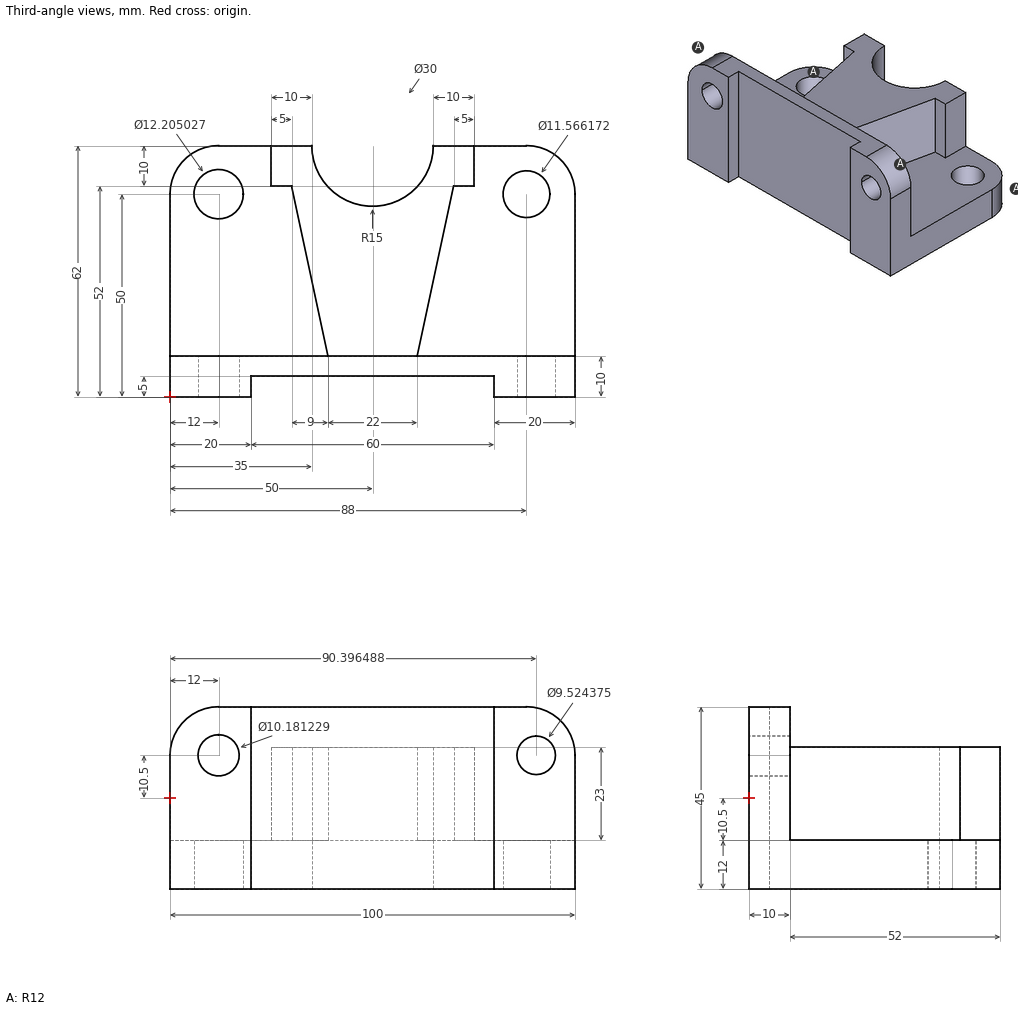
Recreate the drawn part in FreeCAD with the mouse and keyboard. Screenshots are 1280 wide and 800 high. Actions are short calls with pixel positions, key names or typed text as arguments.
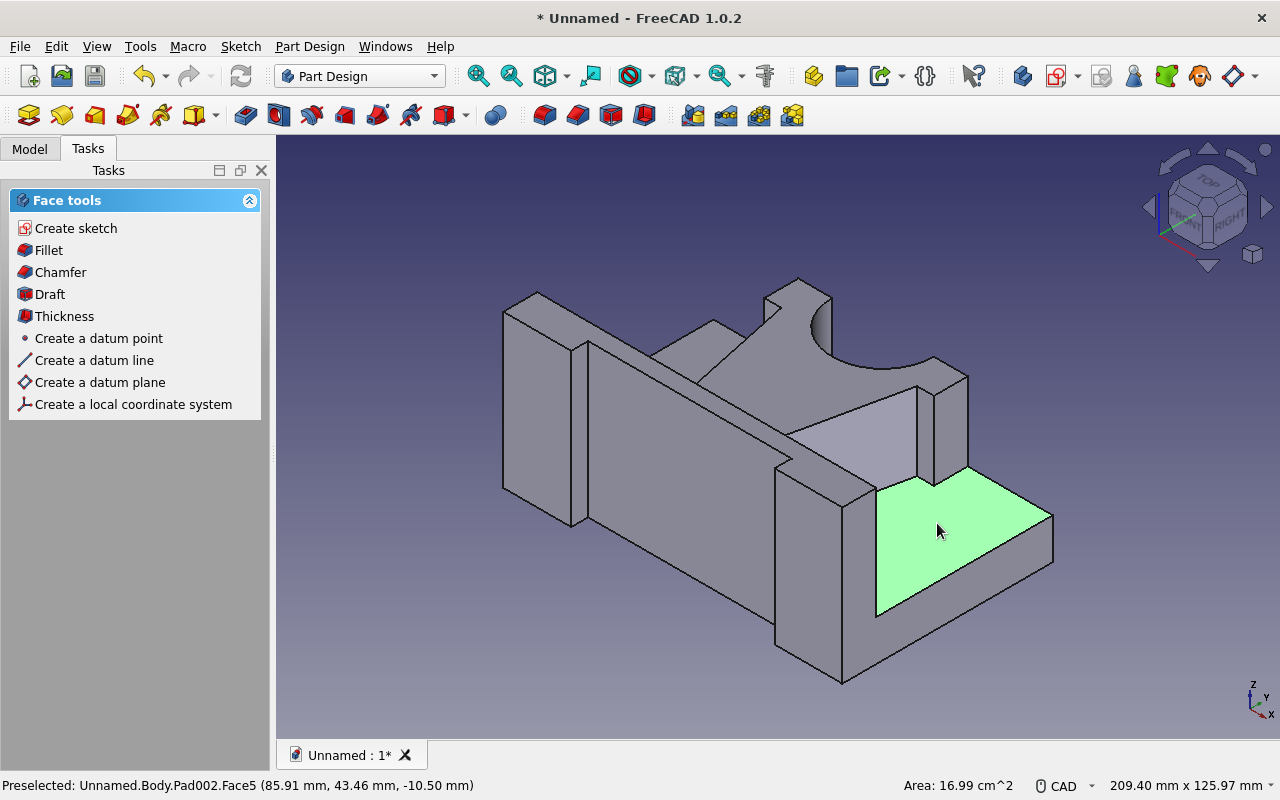
click(1056, 76)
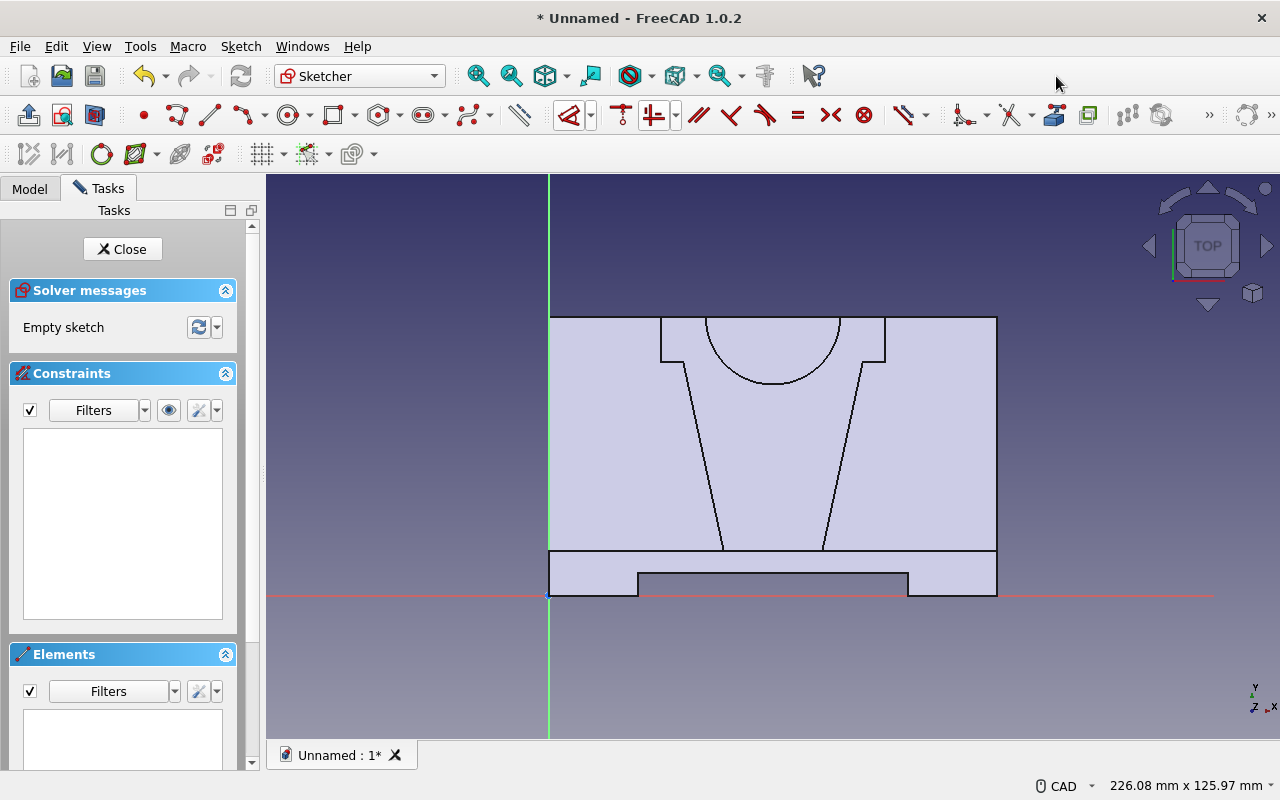
key(g)
key(c)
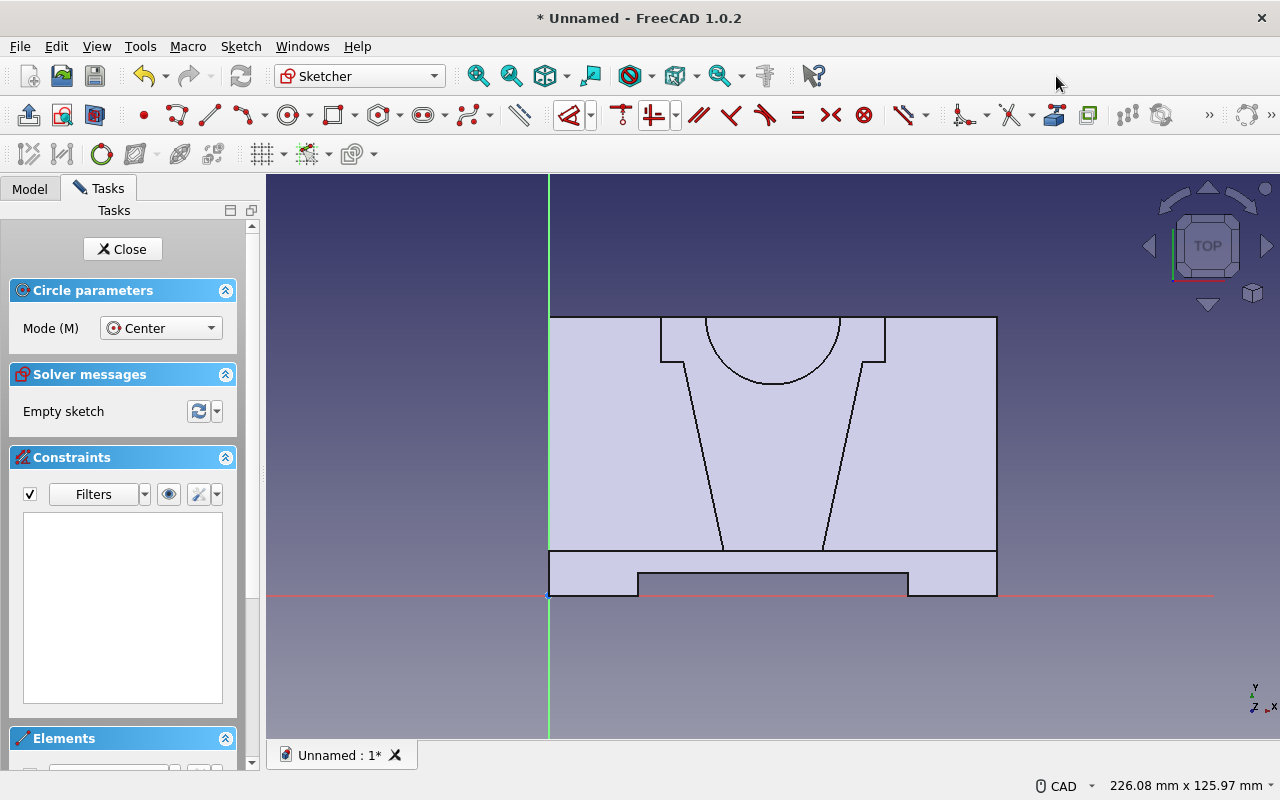
click(773, 317)
click(821, 270)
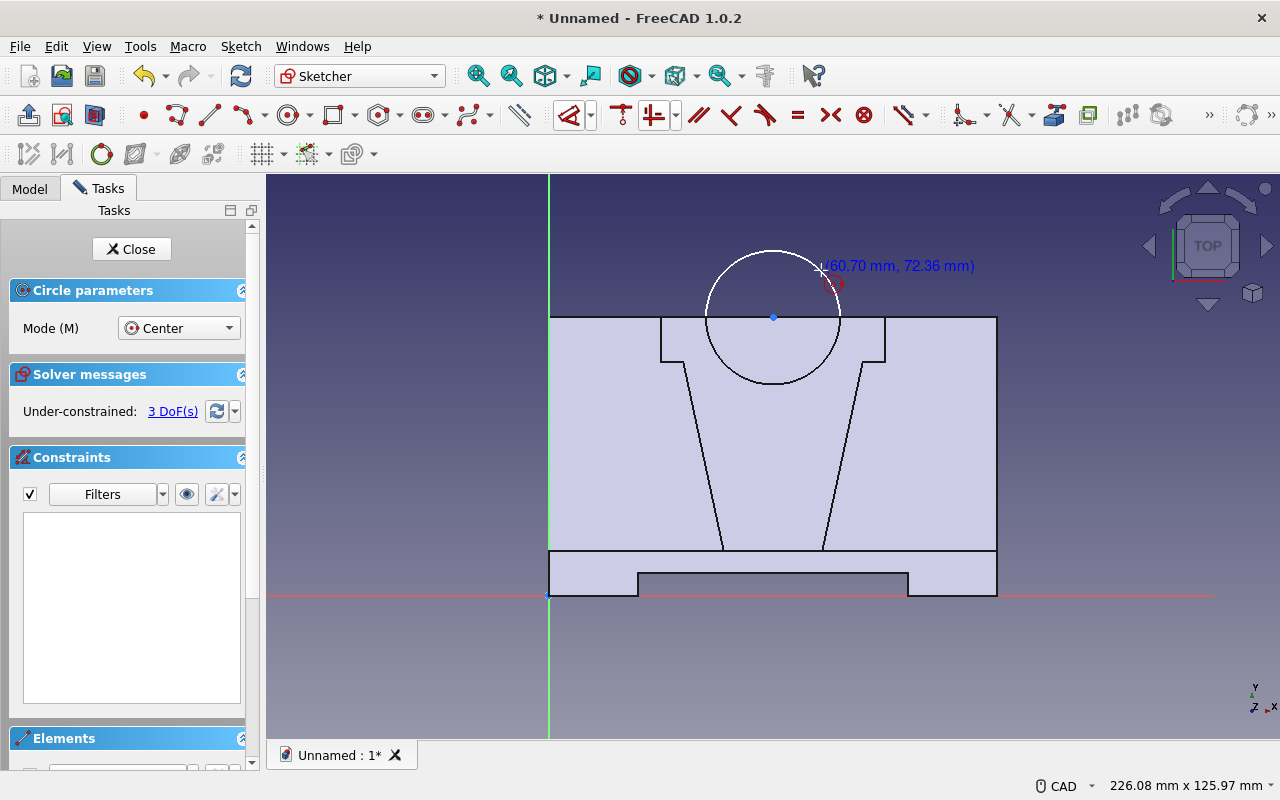
click(603, 371)
click(622, 352)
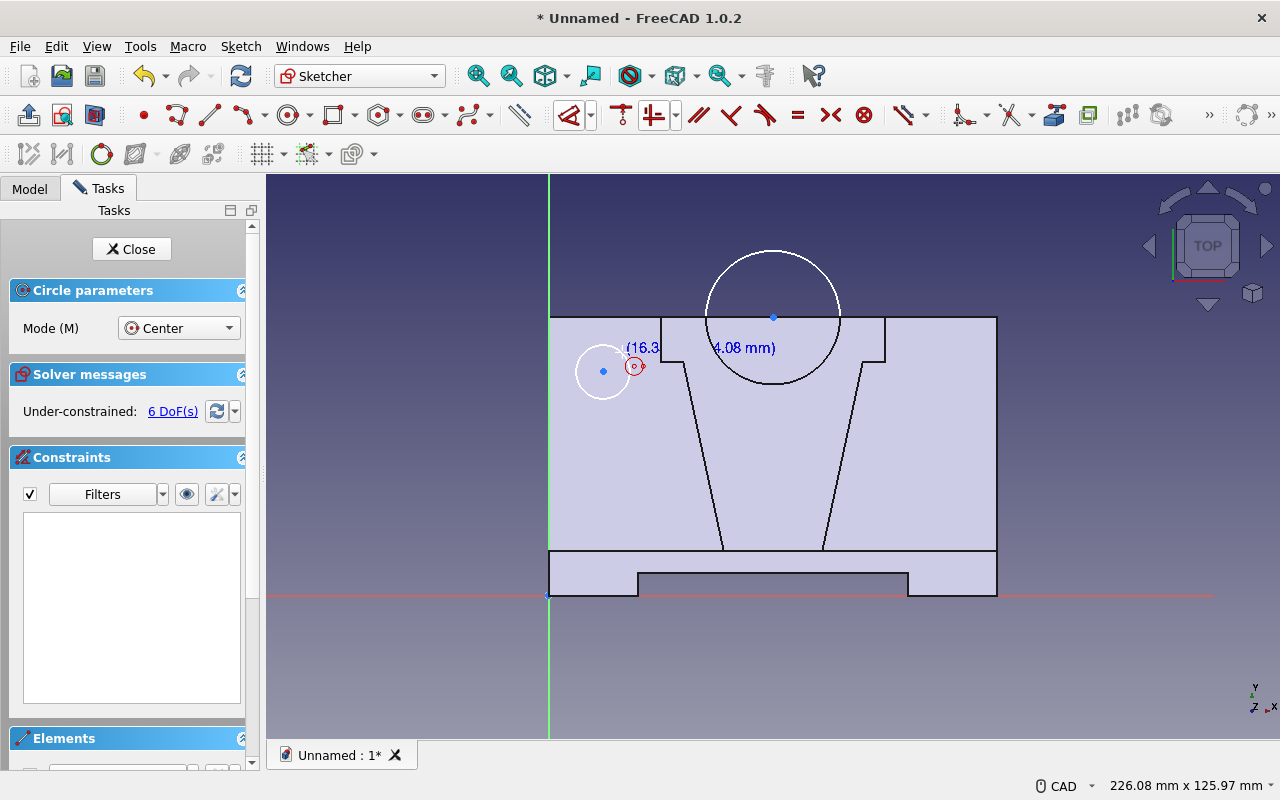
click(943, 371)
click(962, 353)
key(Escape)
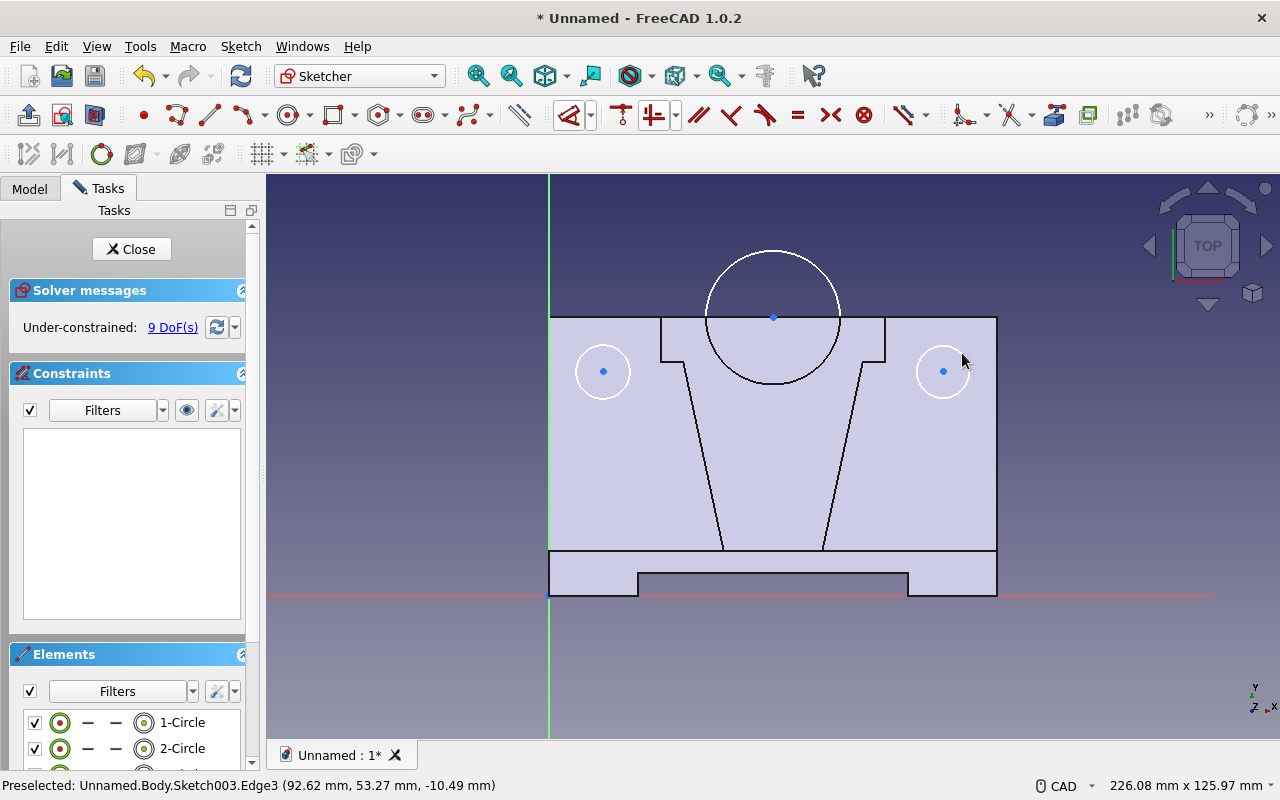
click(603, 372)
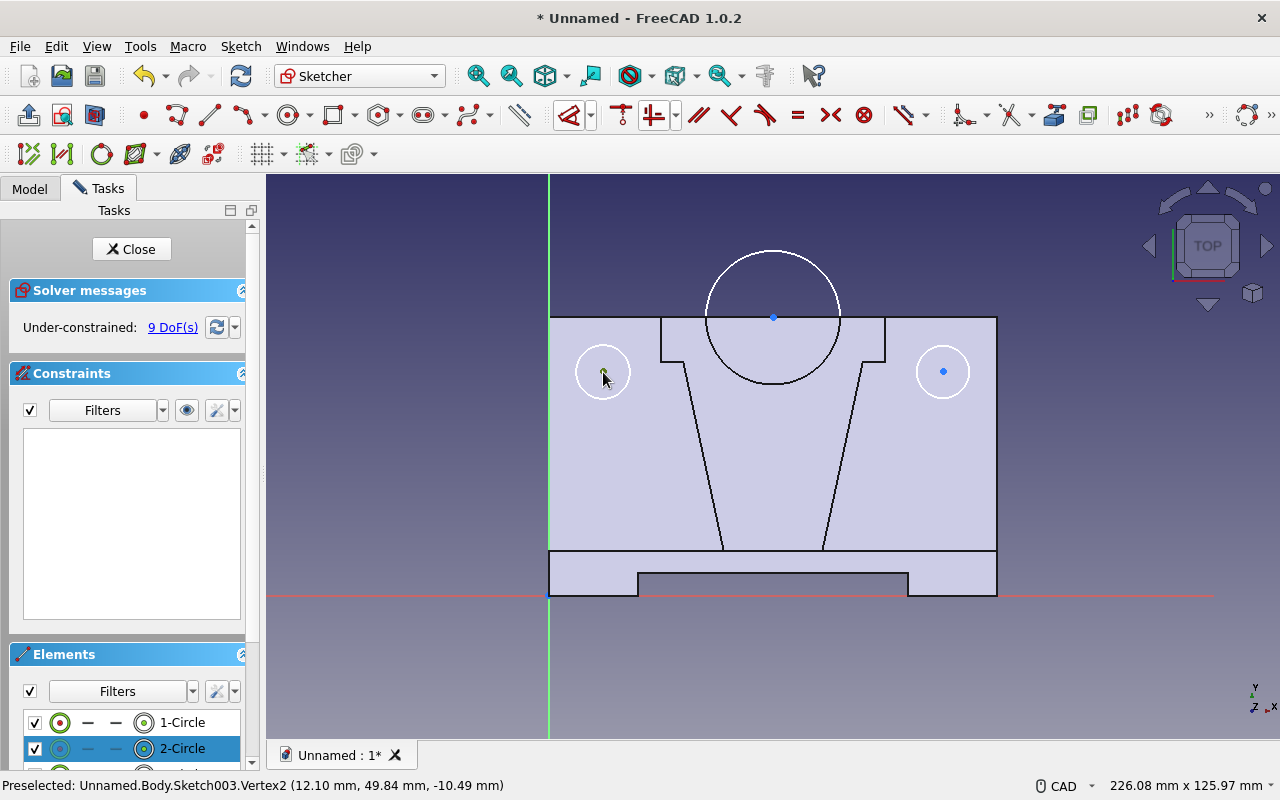
click(943, 372)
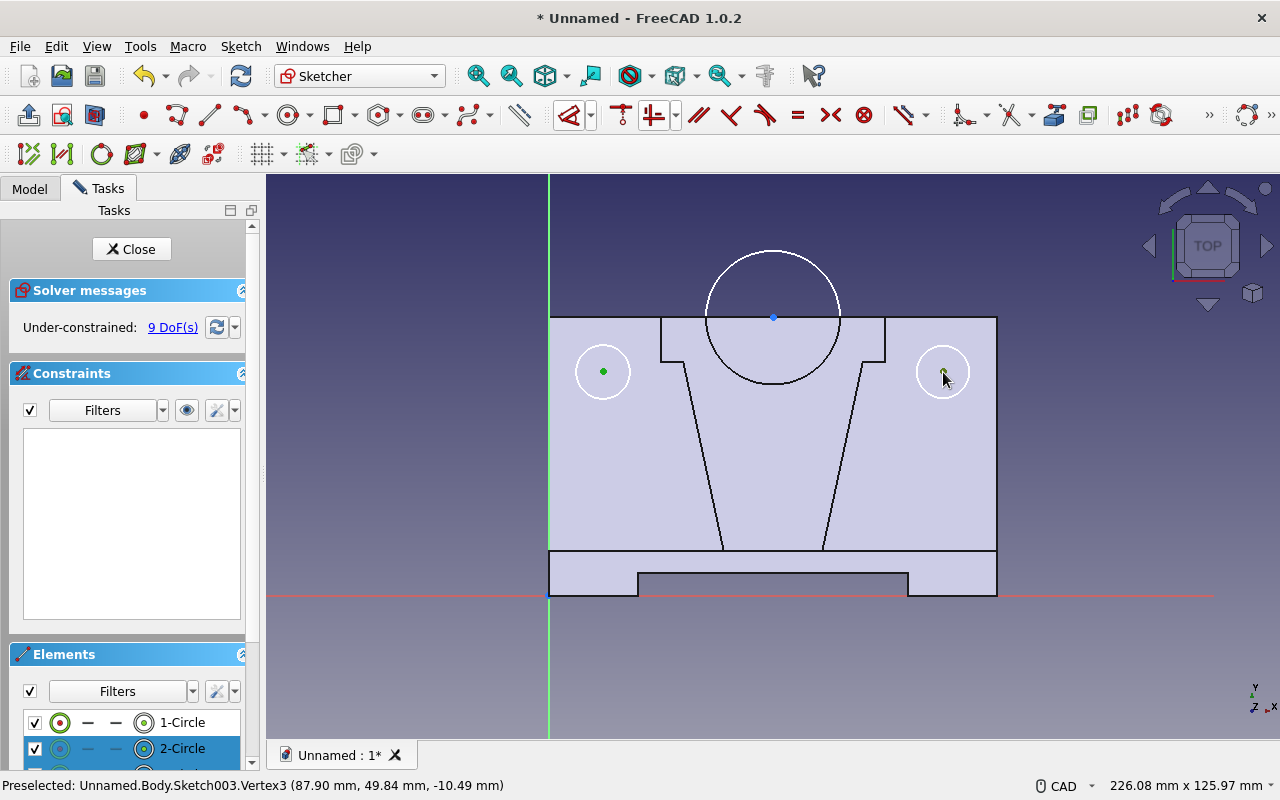
key(h)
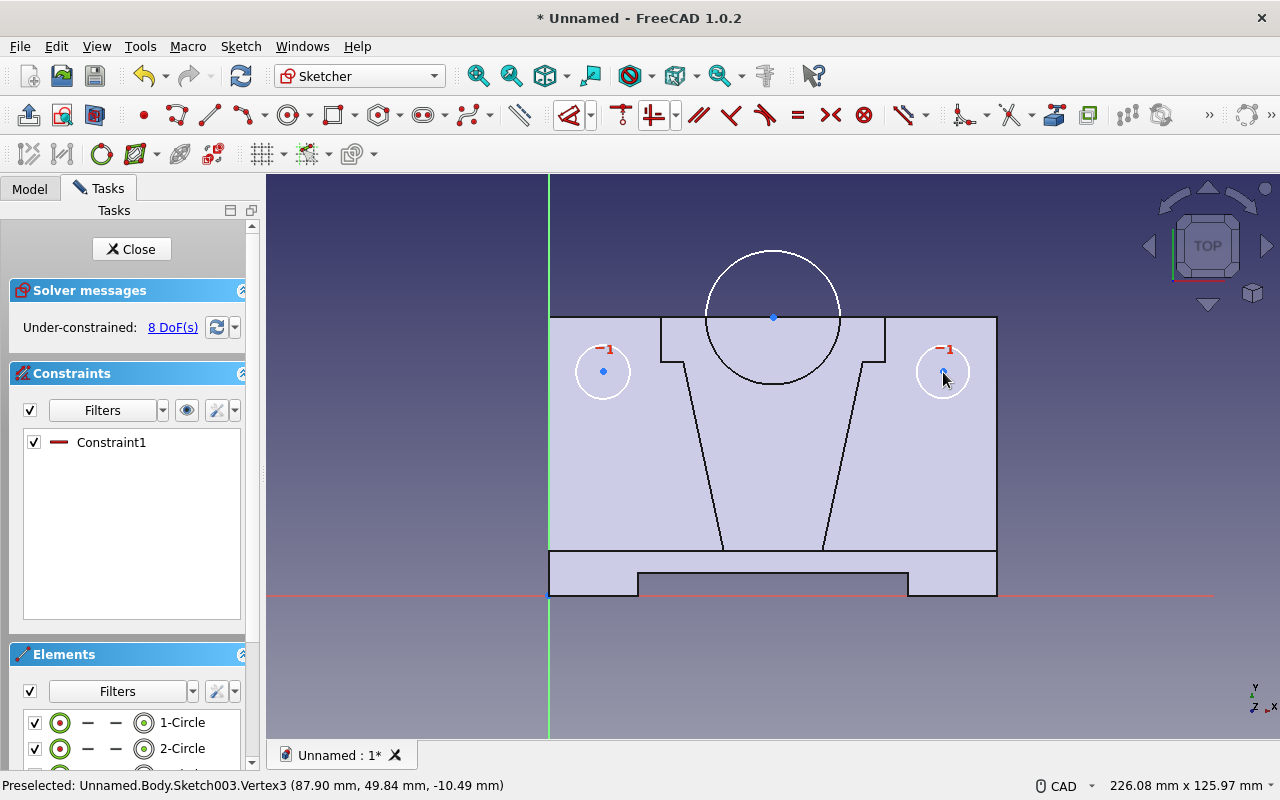
click(820, 270)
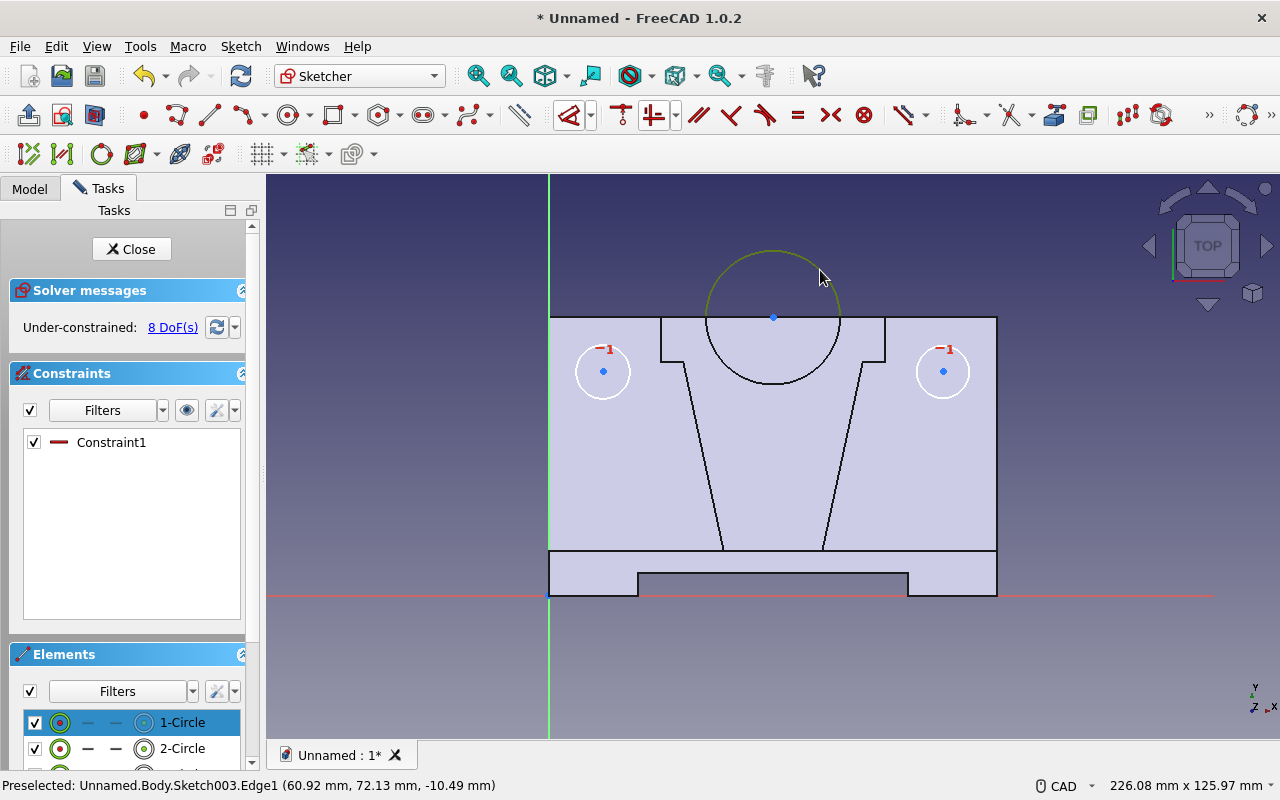
key(k)
key(o)